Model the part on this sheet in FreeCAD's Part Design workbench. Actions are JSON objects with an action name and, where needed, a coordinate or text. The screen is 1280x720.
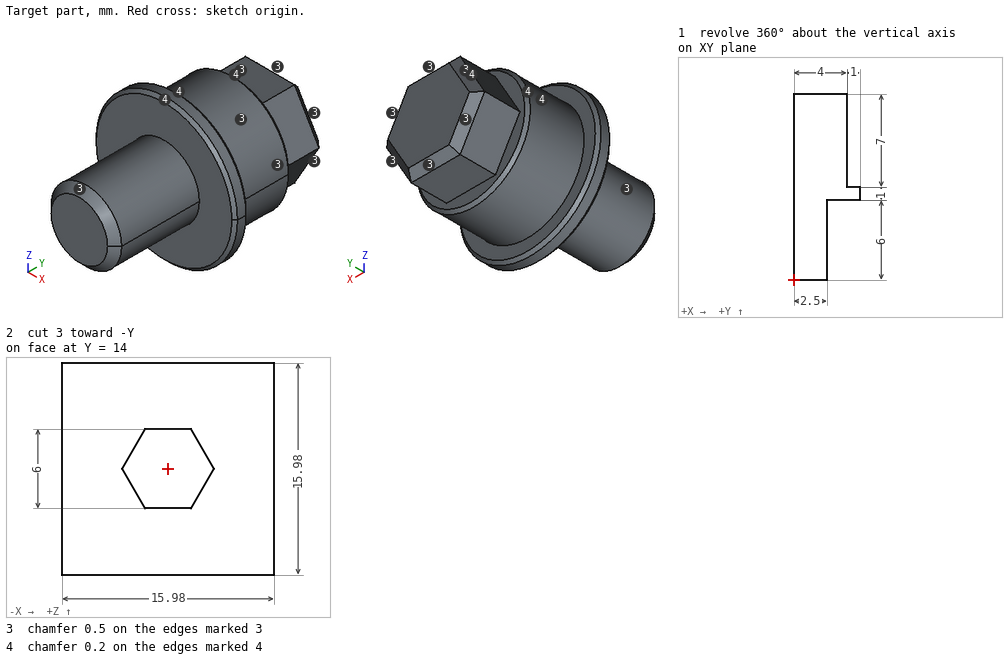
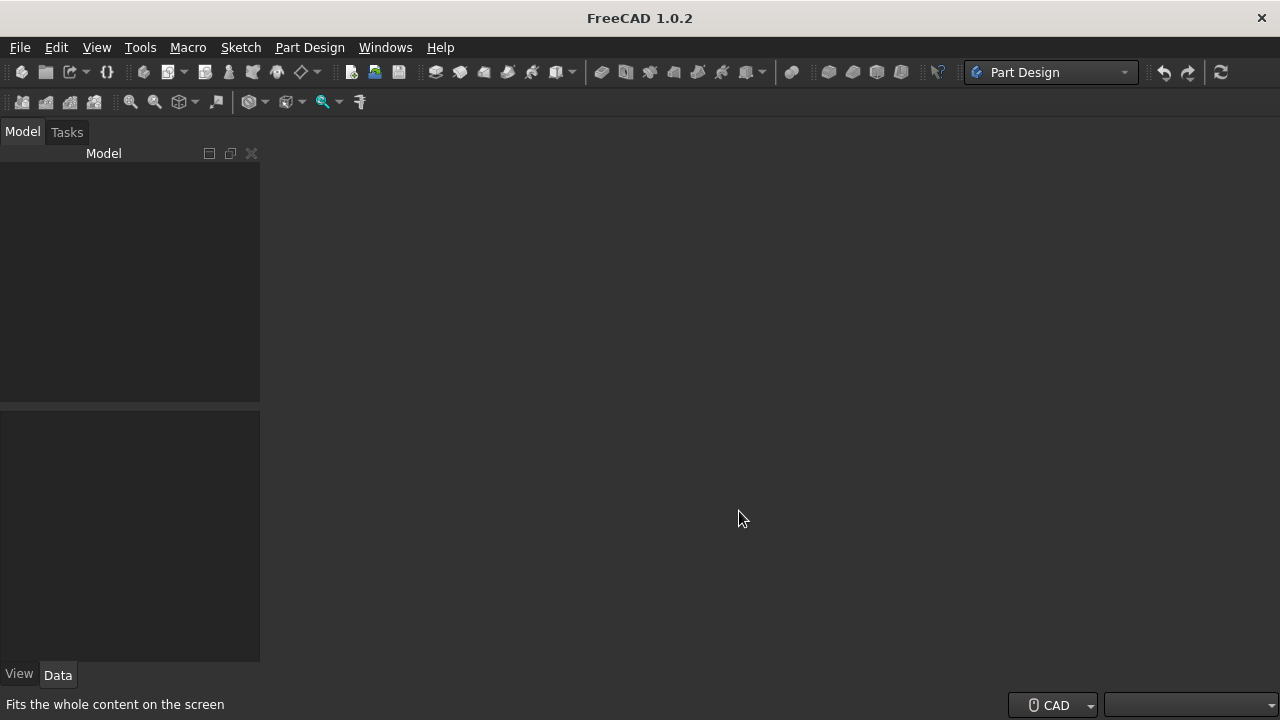
{"action": "left_click", "coordinate": [352, 72]}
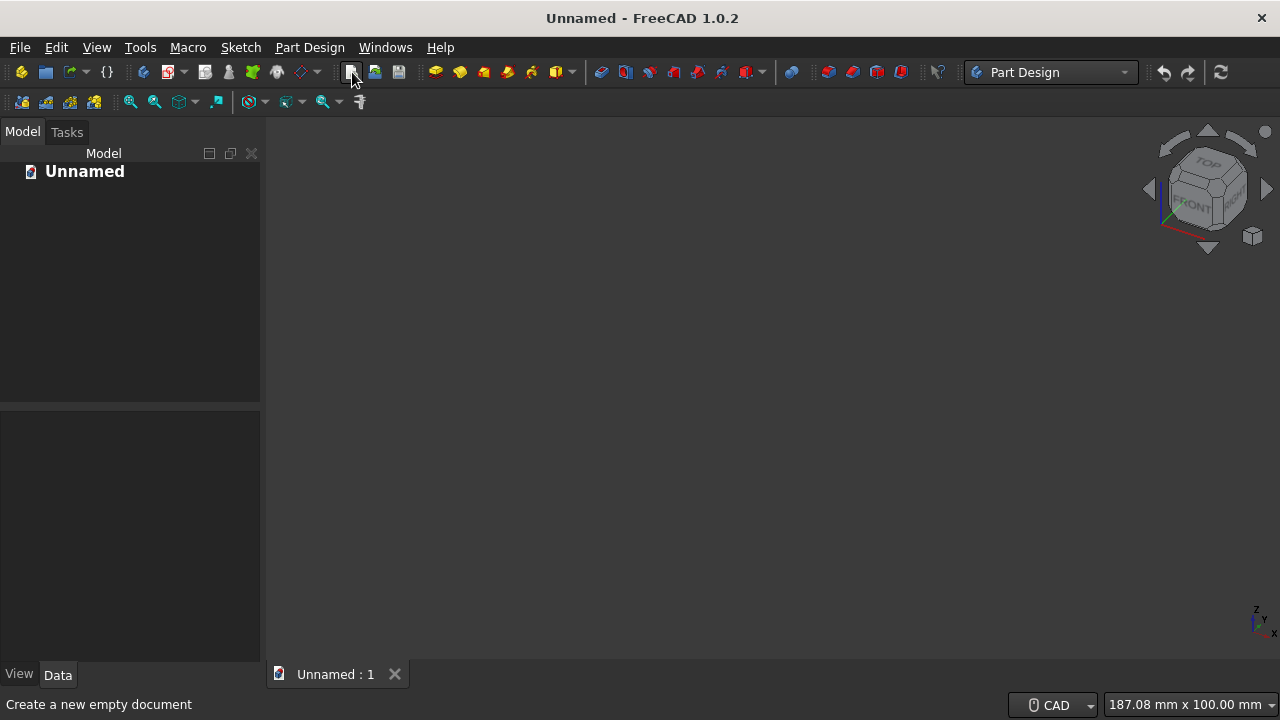
{"action": "left_click", "coordinate": [168, 72]}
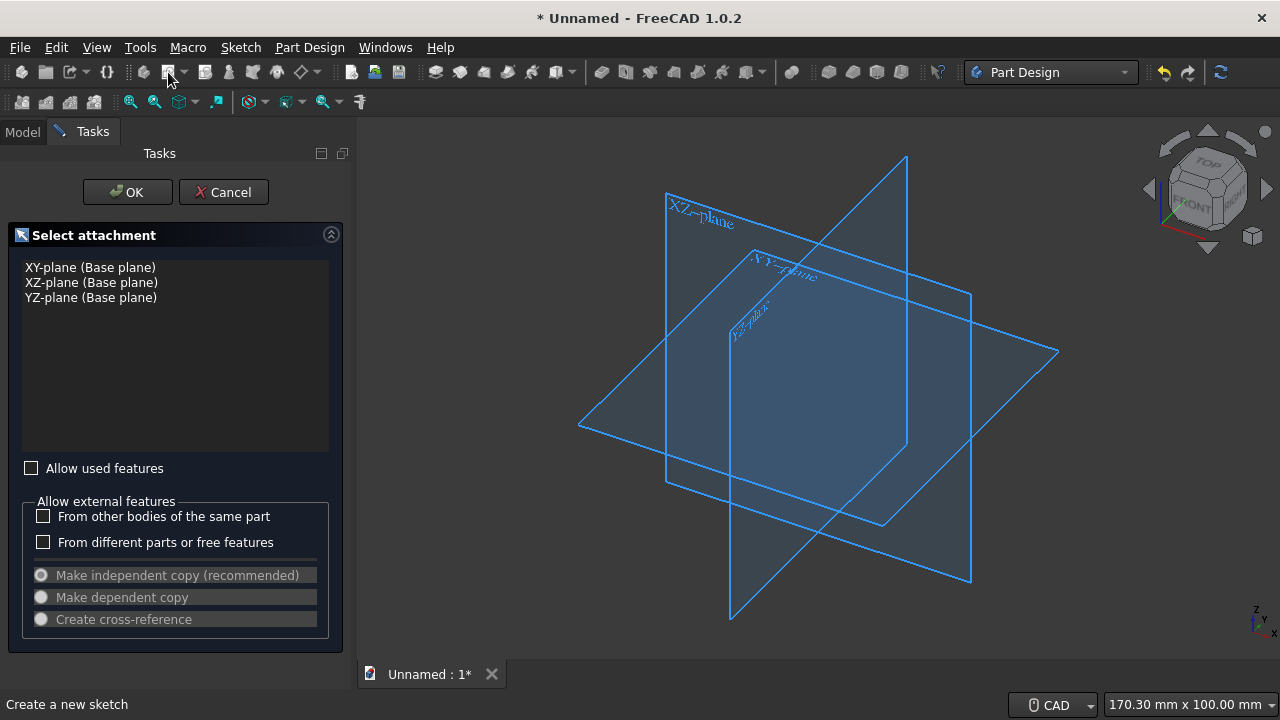
{"action": "left_click", "coordinate": [82, 268]}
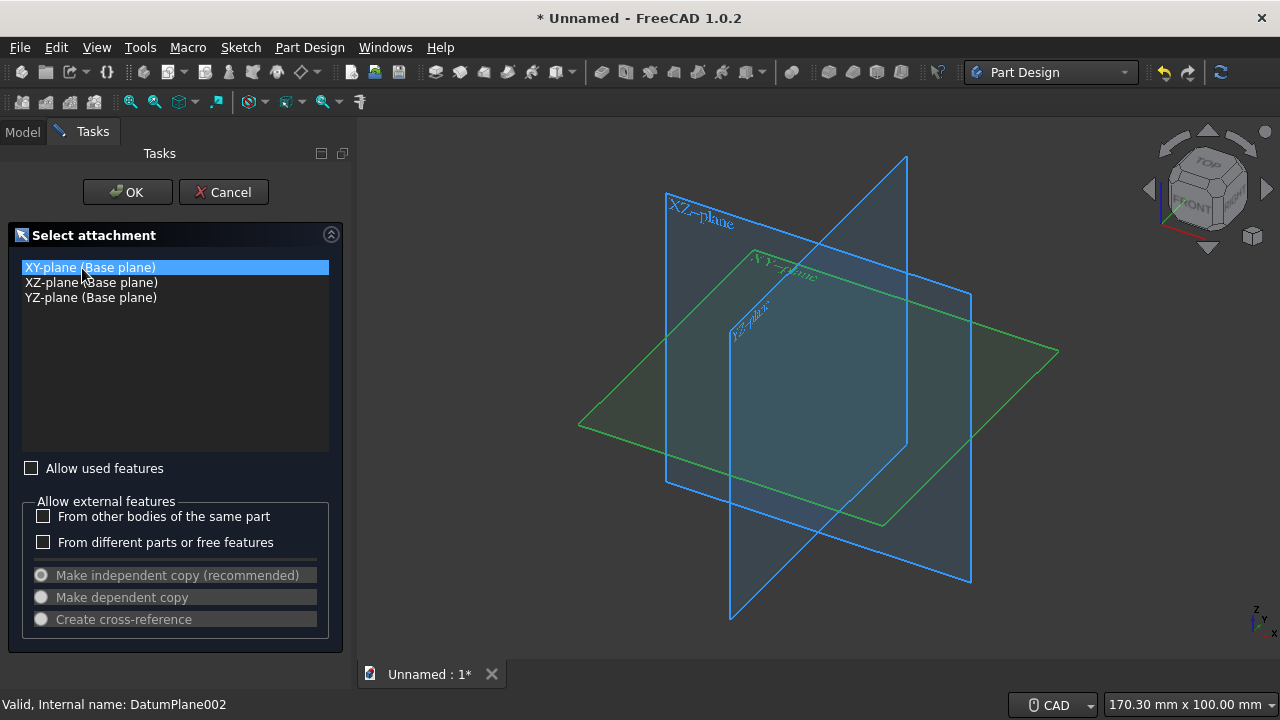
{"action": "left_click", "coordinate": [128, 192]}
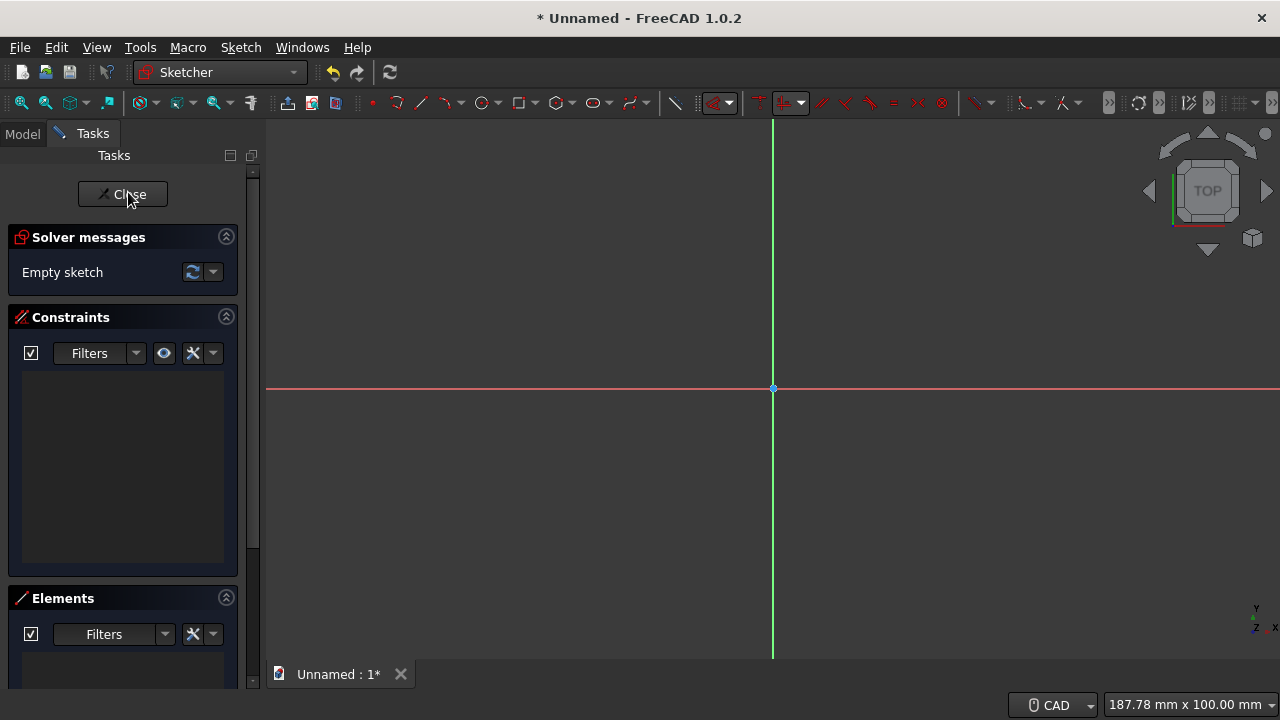
{"action": "scroll", "coordinate": [807, 342], "scroll_direction": "up", "scroll_amount": 8}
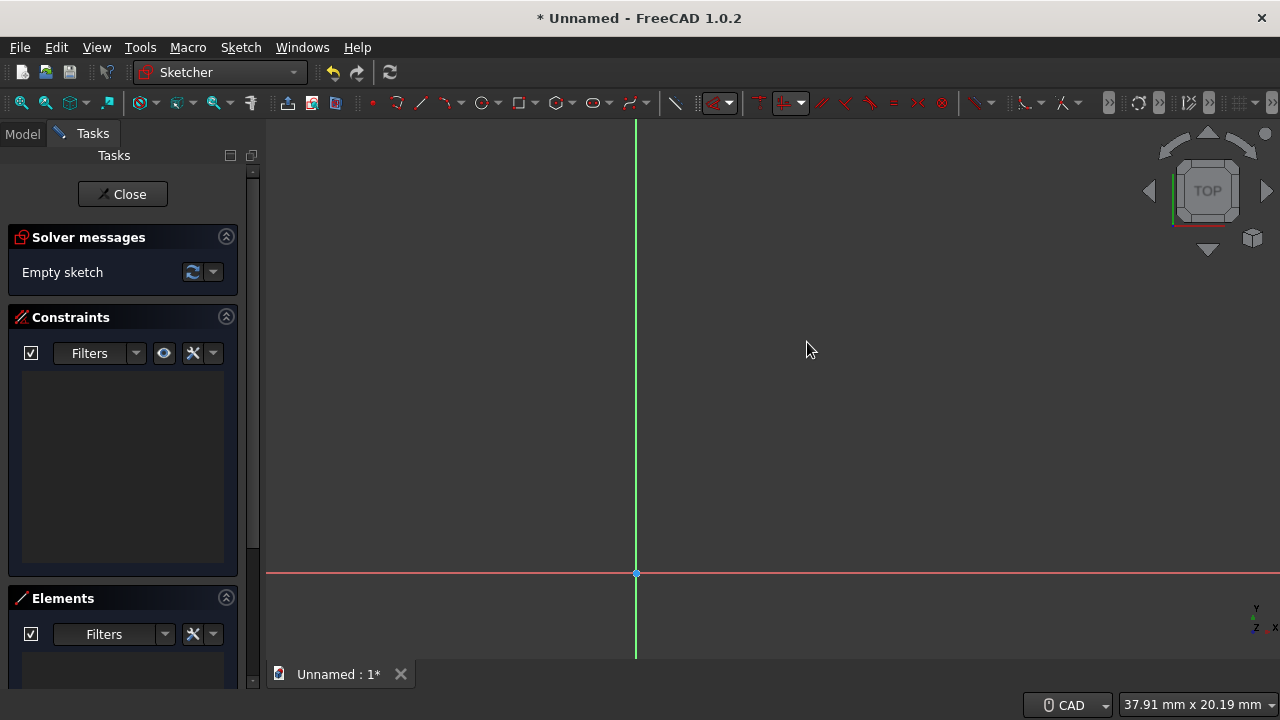
{"action": "left_click", "coordinate": [398, 104]}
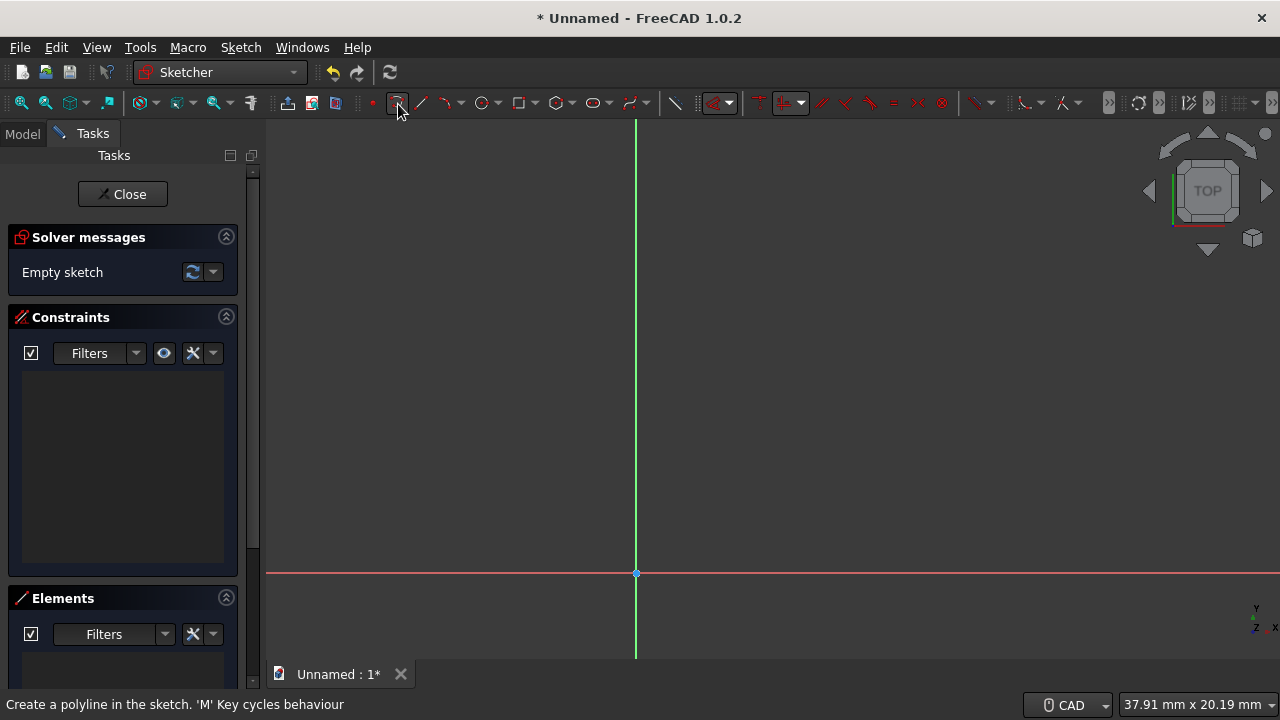
{"action": "left_click", "coordinate": [636, 573]}
{"action": "left_click", "coordinate": [703, 564]}
{"action": "left_click", "coordinate": [703, 413]}
{"action": "left_click", "coordinate": [770, 413]}
{"action": "left_click", "coordinate": [770, 386]}
{"action": "left_click", "coordinate": [743, 386]}
{"action": "left_click", "coordinate": [743, 199]}
{"action": "left_click", "coordinate": [645, 199]}
{"action": "left_click", "coordinate": [636, 573]}
{"action": "key", "text": "Escape"}
{"action": "key", "text": "Escape"}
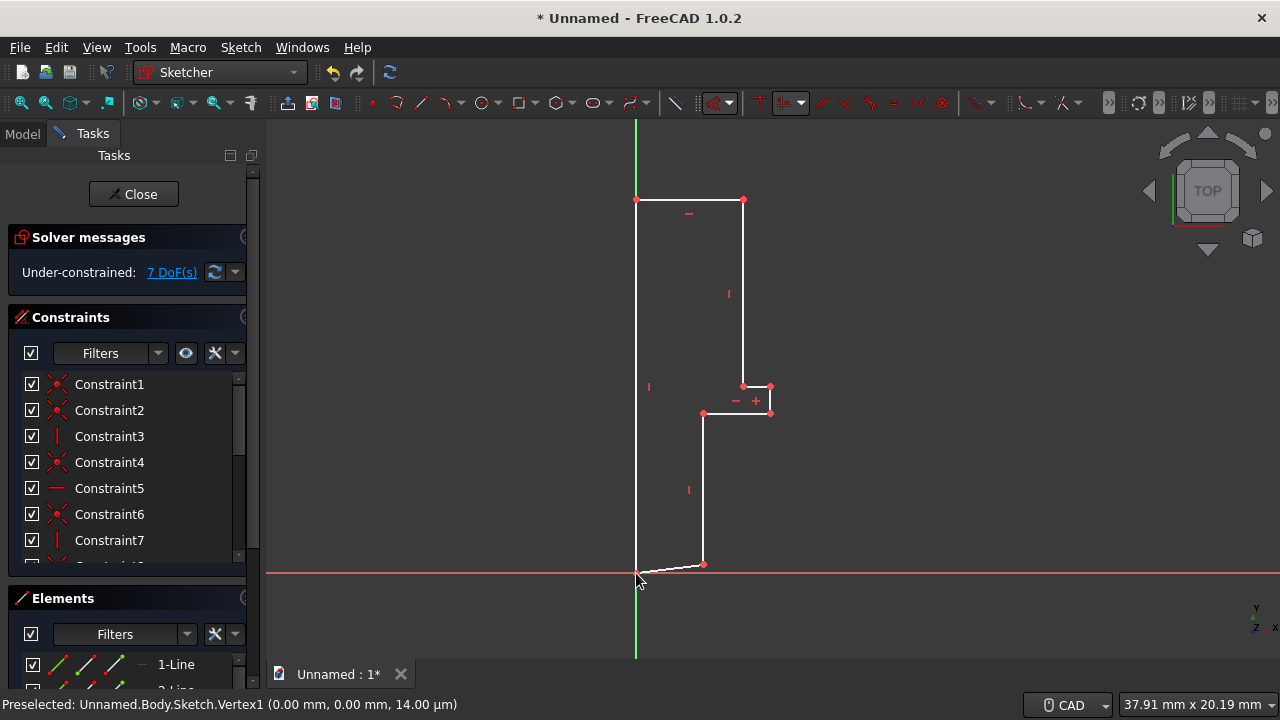
{"action": "left_click", "coordinate": [656, 571]}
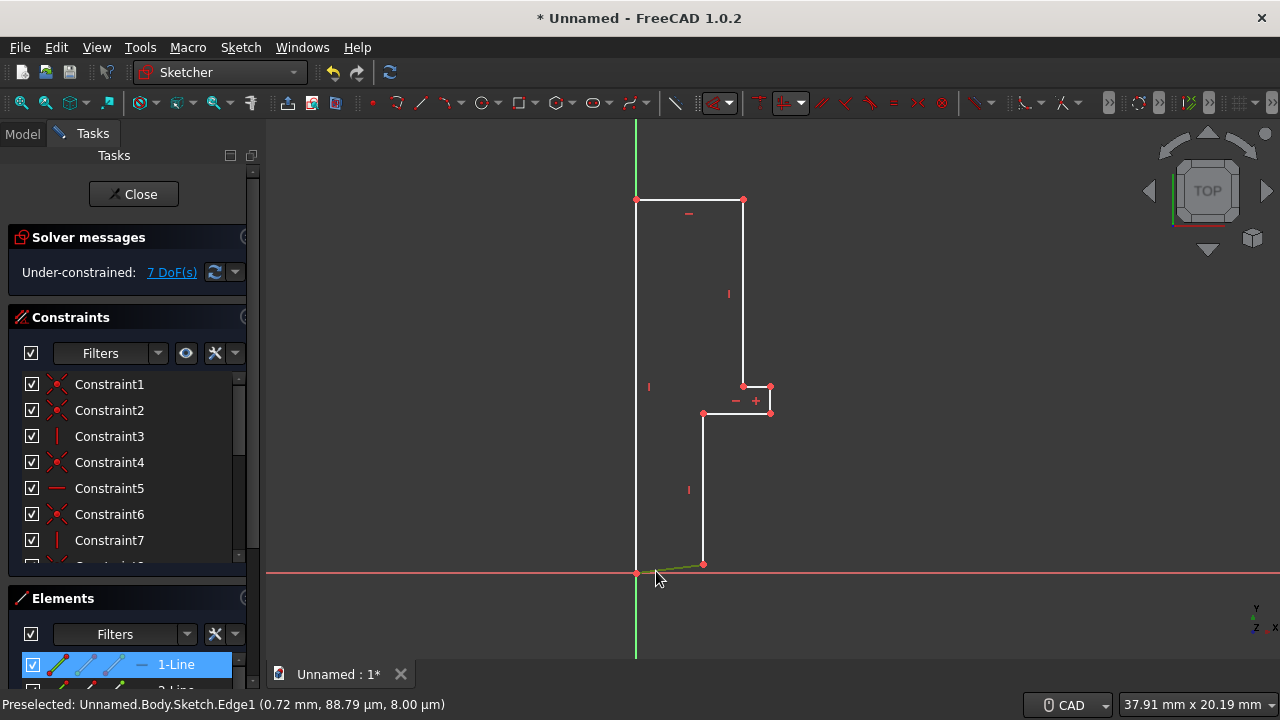
{"action": "left_click", "coordinate": [804, 104]}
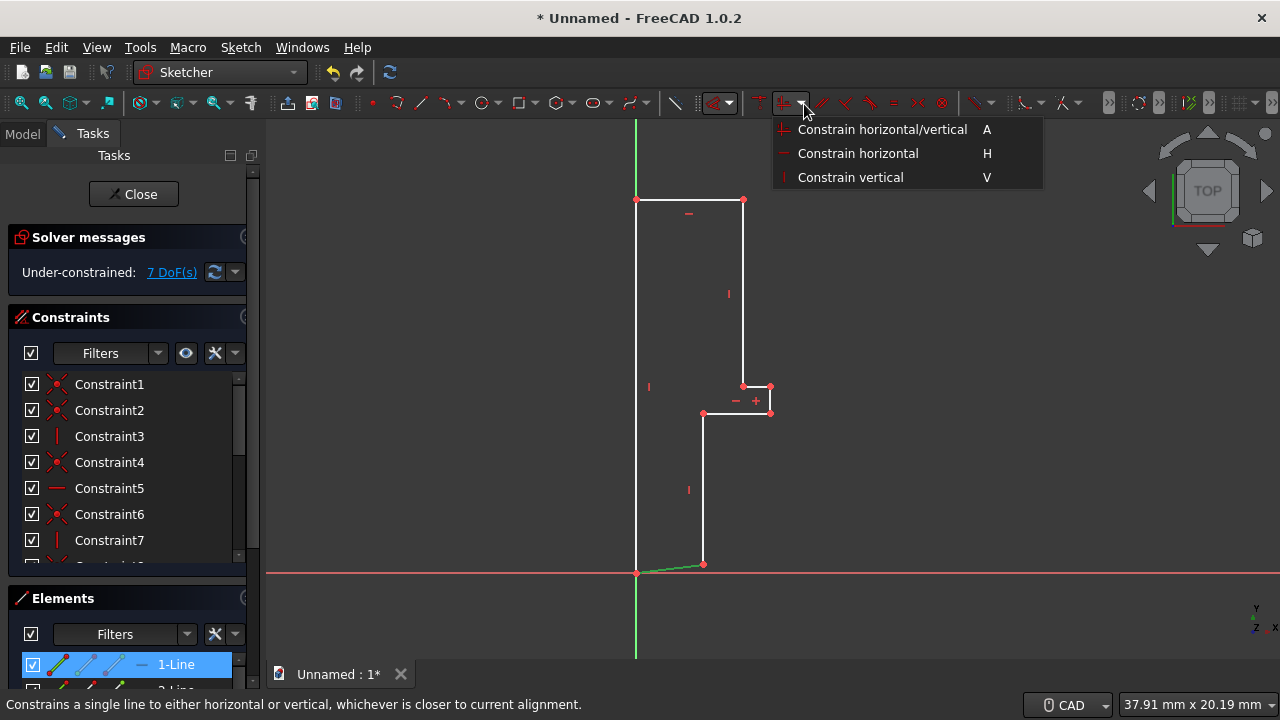
{"action": "left_click", "coordinate": [908, 153]}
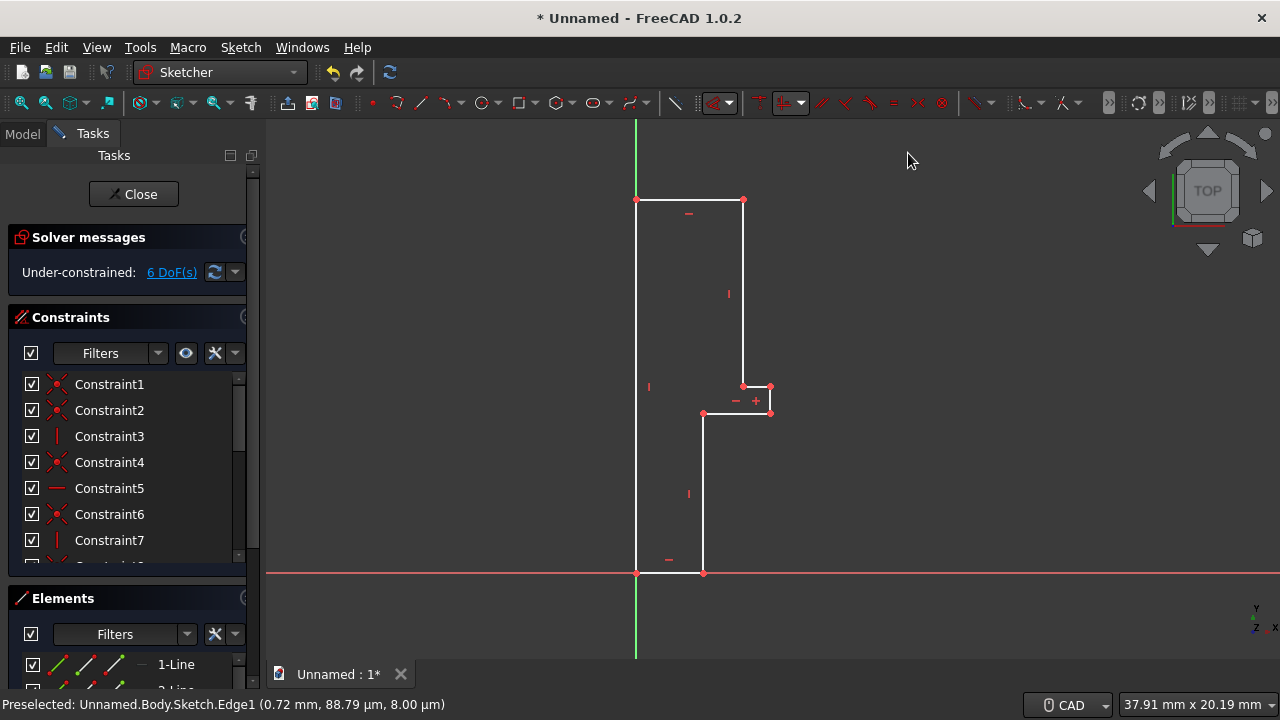
{"action": "left_click", "coordinate": [714, 104]}